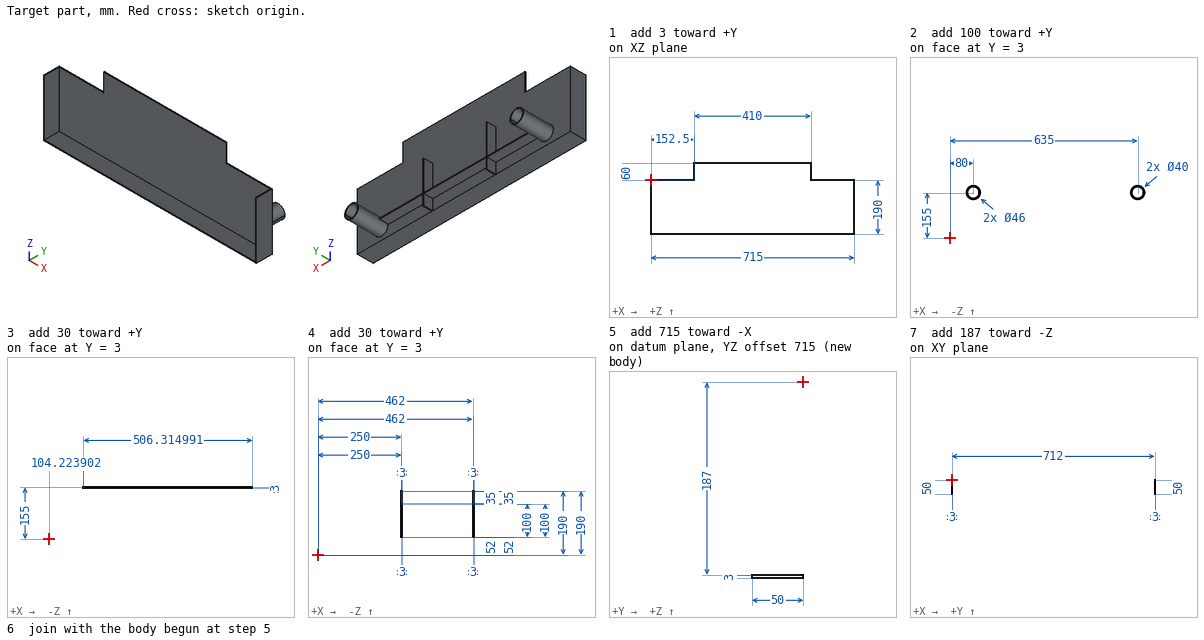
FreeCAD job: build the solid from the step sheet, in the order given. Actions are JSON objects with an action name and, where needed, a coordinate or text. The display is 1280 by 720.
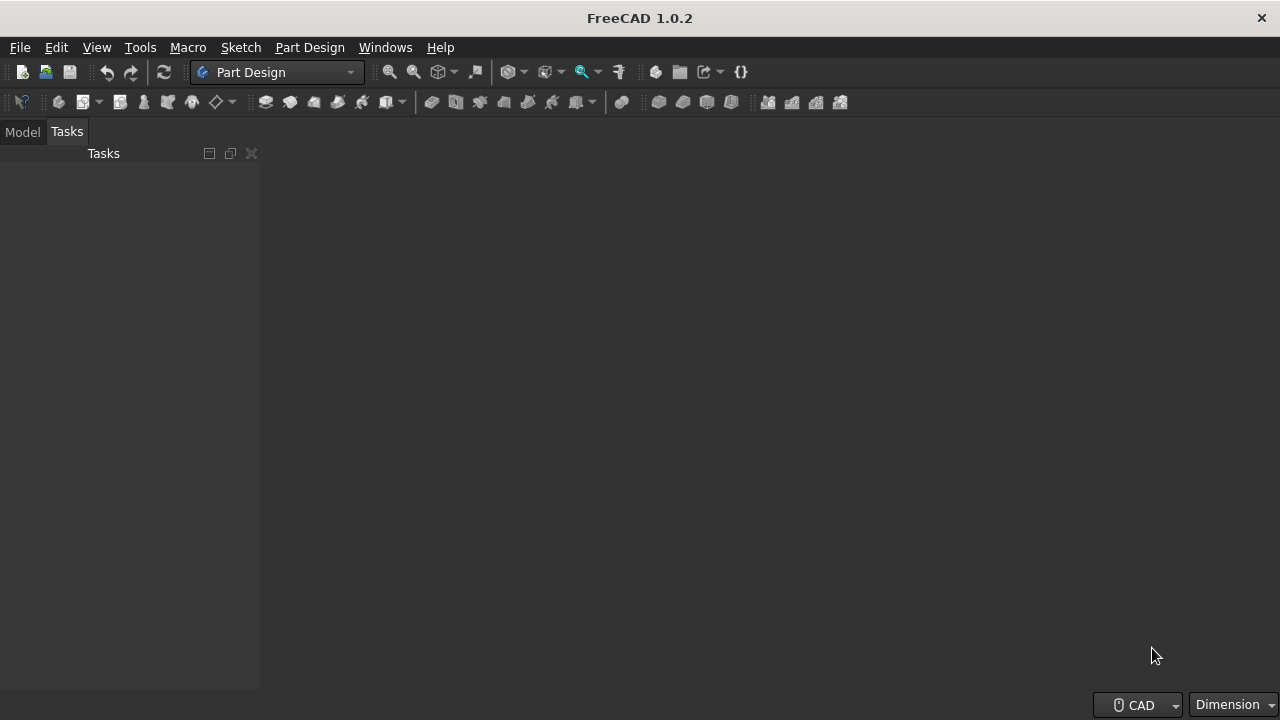
{"action": "left_click", "coordinate": [22, 72]}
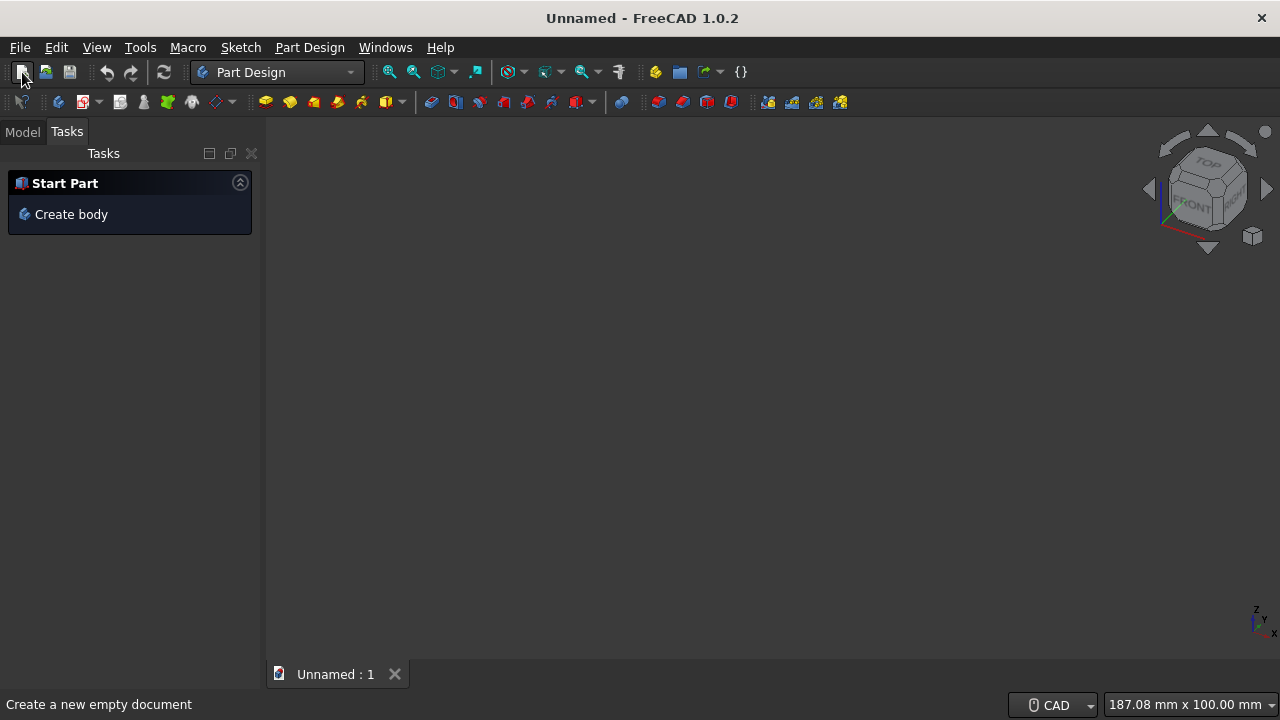
{"action": "left_click", "coordinate": [84, 102]}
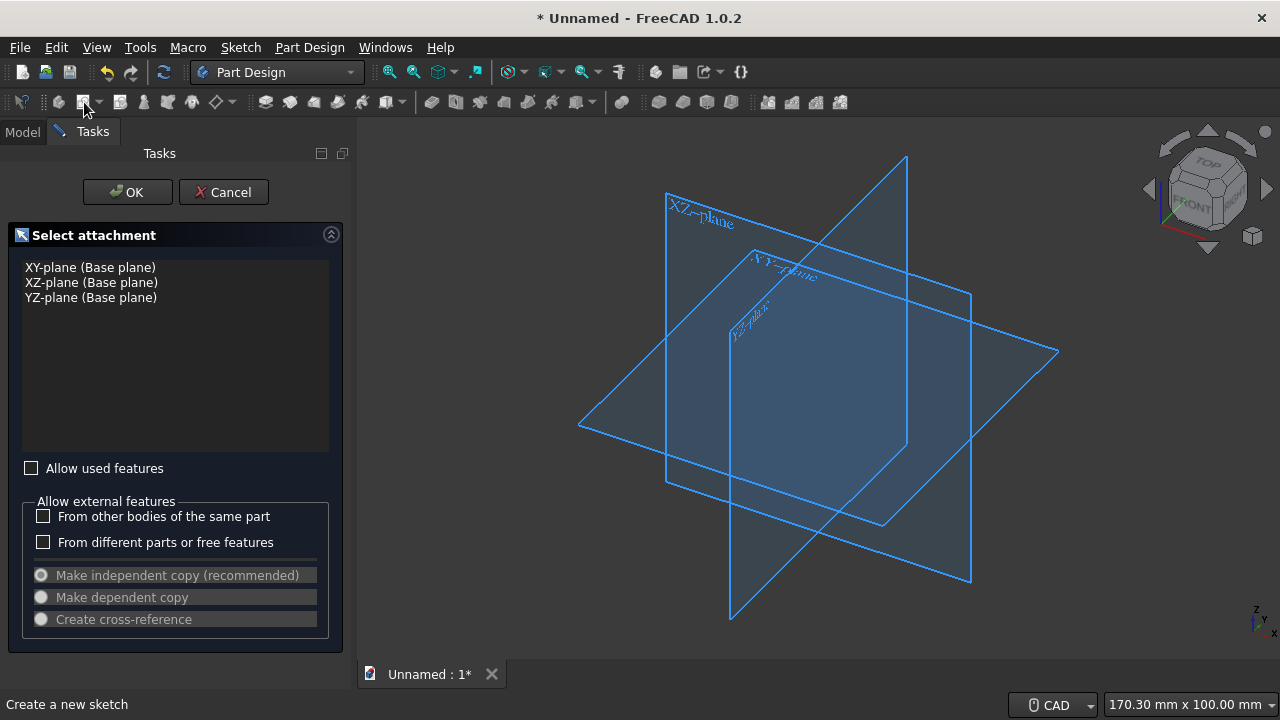
{"action": "left_click", "coordinate": [82, 282]}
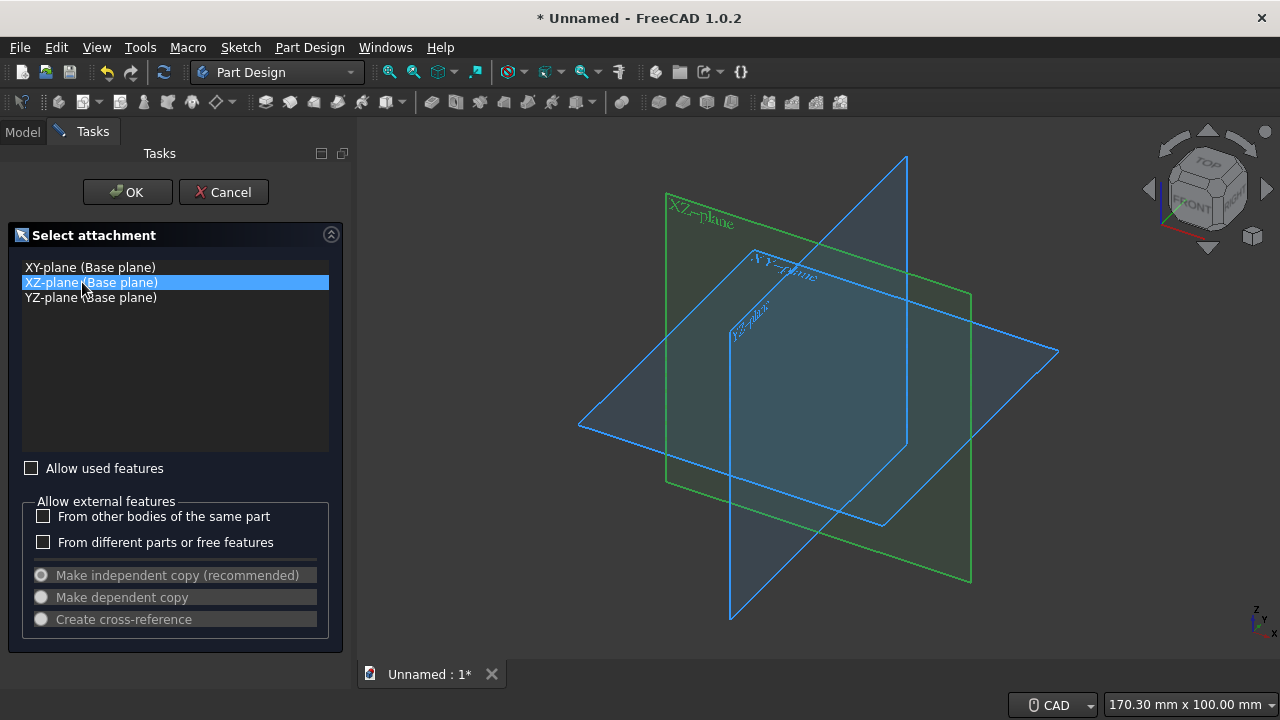
{"action": "left_click", "coordinate": [128, 192]}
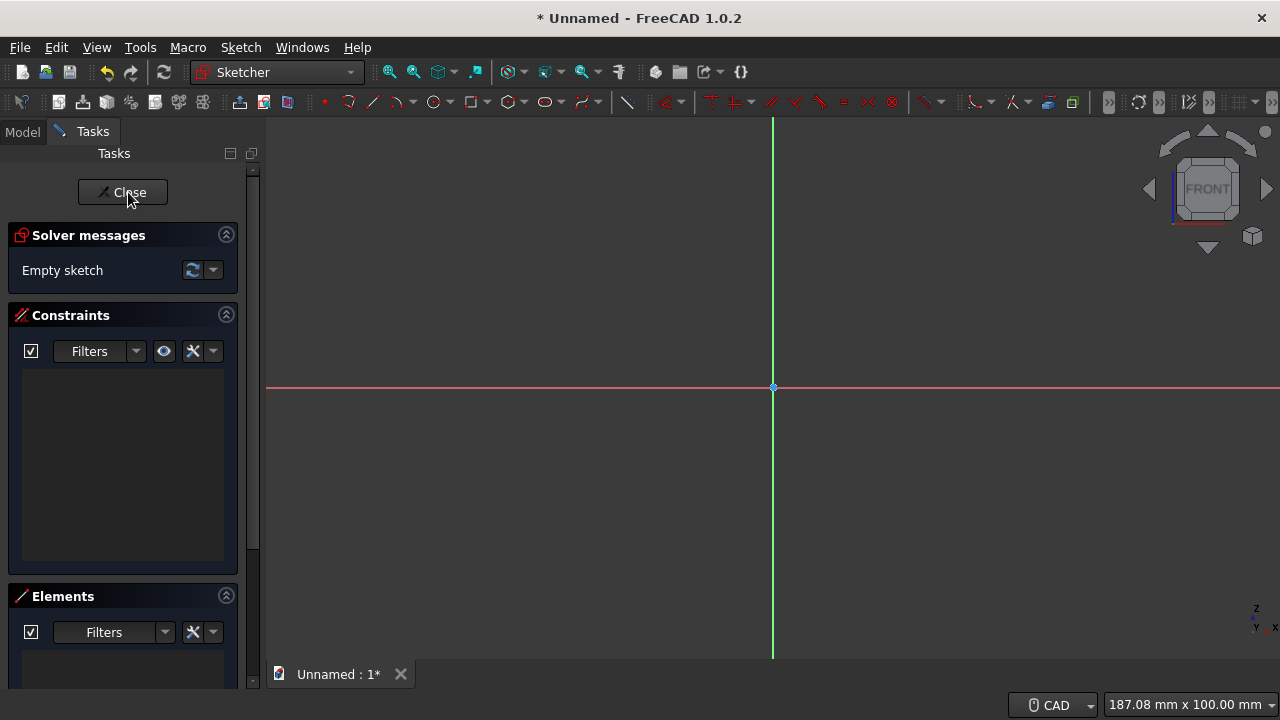
{"action": "scroll", "coordinate": [391, 333], "scroll_direction": "down", "scroll_amount": 10}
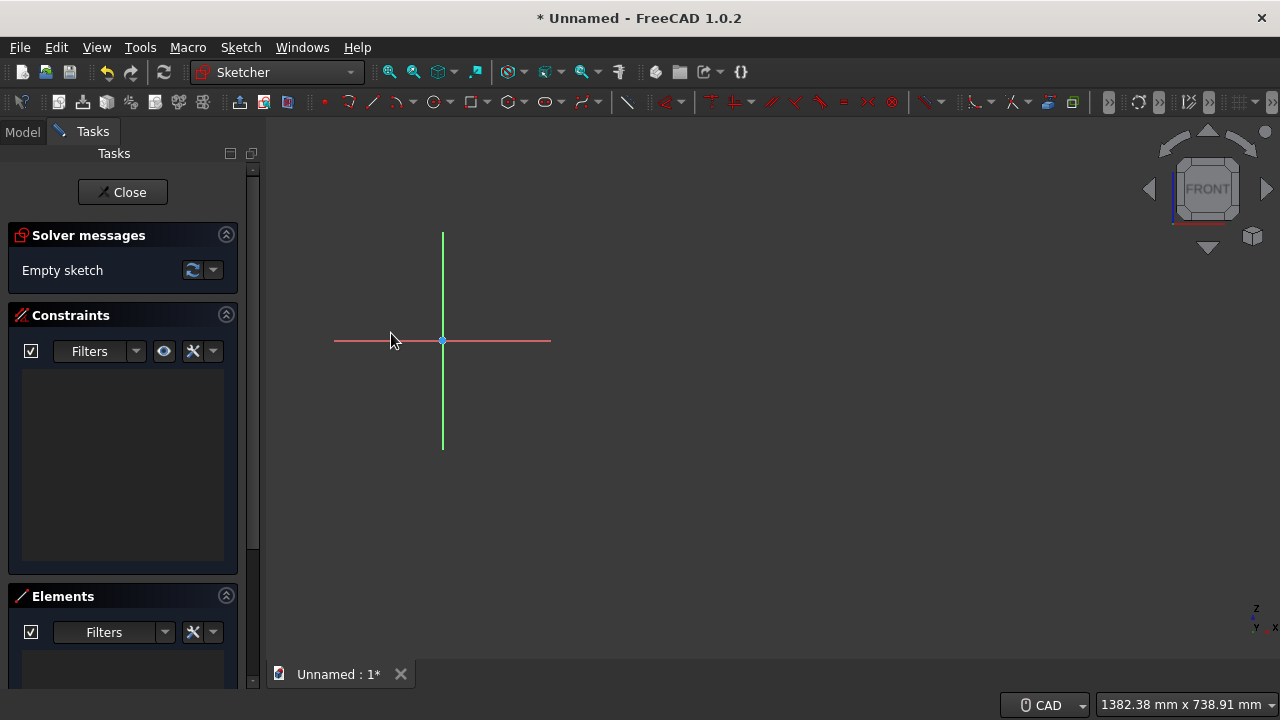
{"action": "key", "text": "g m"}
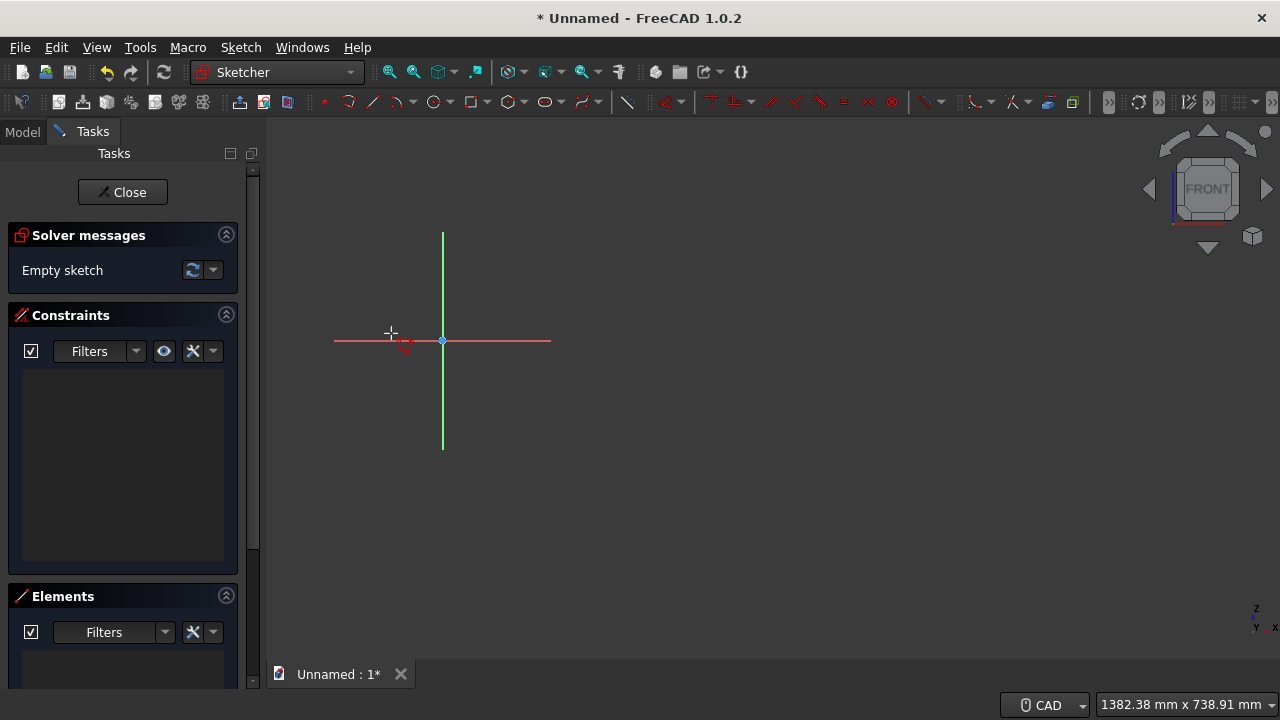
{"action": "left_click", "coordinate": [443, 341]}
{"action": "left_click", "coordinate": [555, 350]}
{"action": "left_click", "coordinate": [555, 297]}
{"action": "left_click", "coordinate": [855, 297]}
{"action": "left_click", "coordinate": [855, 341]}
{"action": "left_click", "coordinate": [967, 350]}
{"action": "left_click", "coordinate": [967, 480]}
{"action": "left_click", "coordinate": [452, 480]}
{"action": "left_click", "coordinate": [443, 341]}
{"action": "key", "text": "Escape"}
{"action": "key", "text": "Escape"}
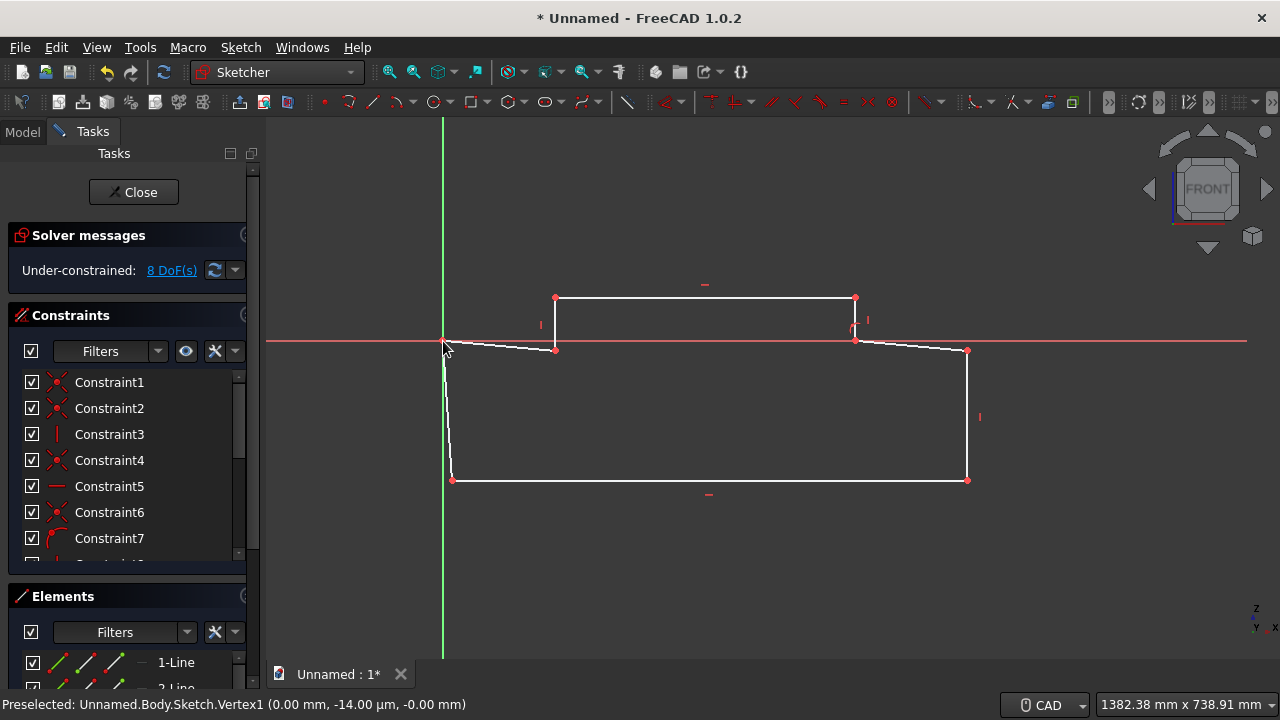
{"action": "left_click", "coordinate": [476, 344]}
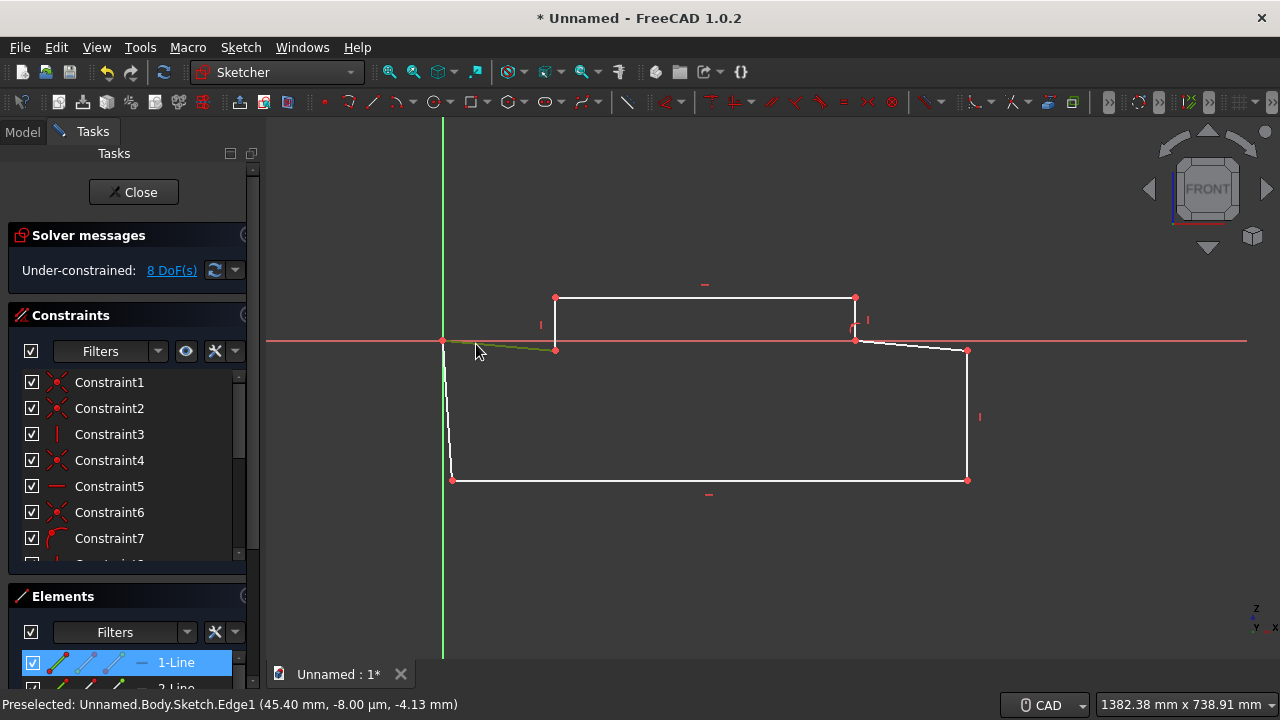
{"action": "left_click", "coordinate": [754, 102]}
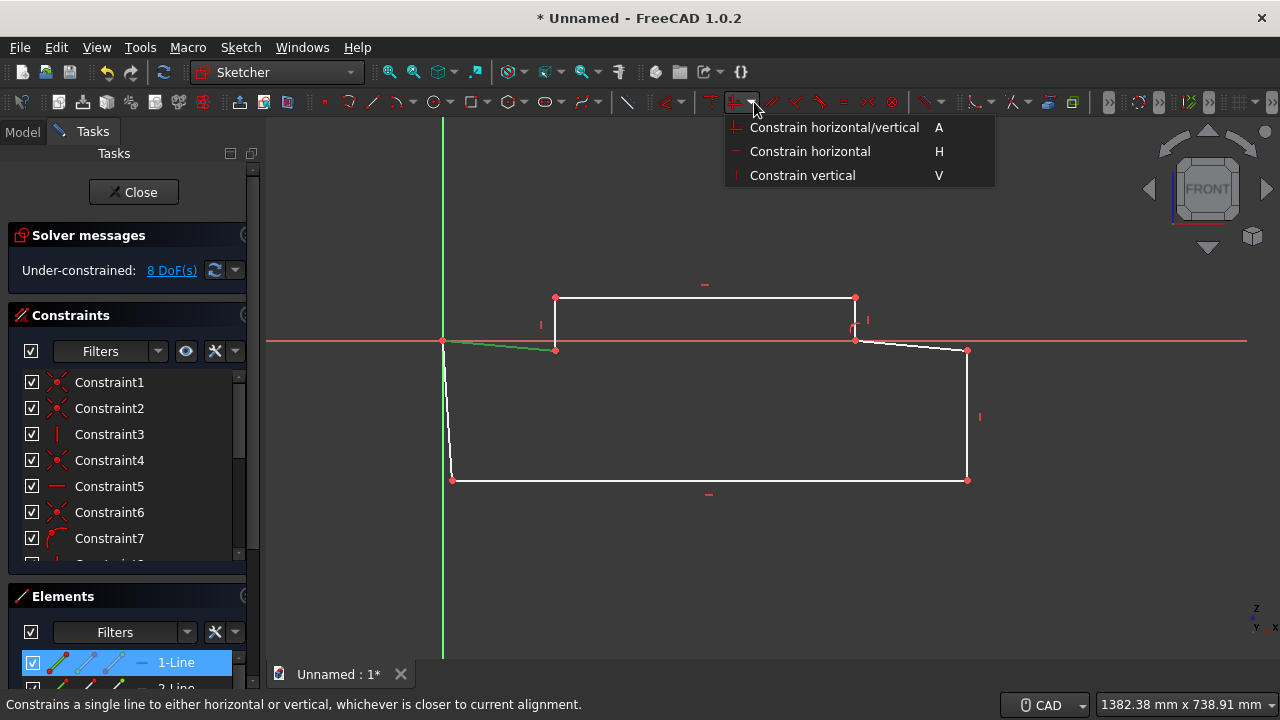
{"action": "left_click", "coordinate": [860, 151]}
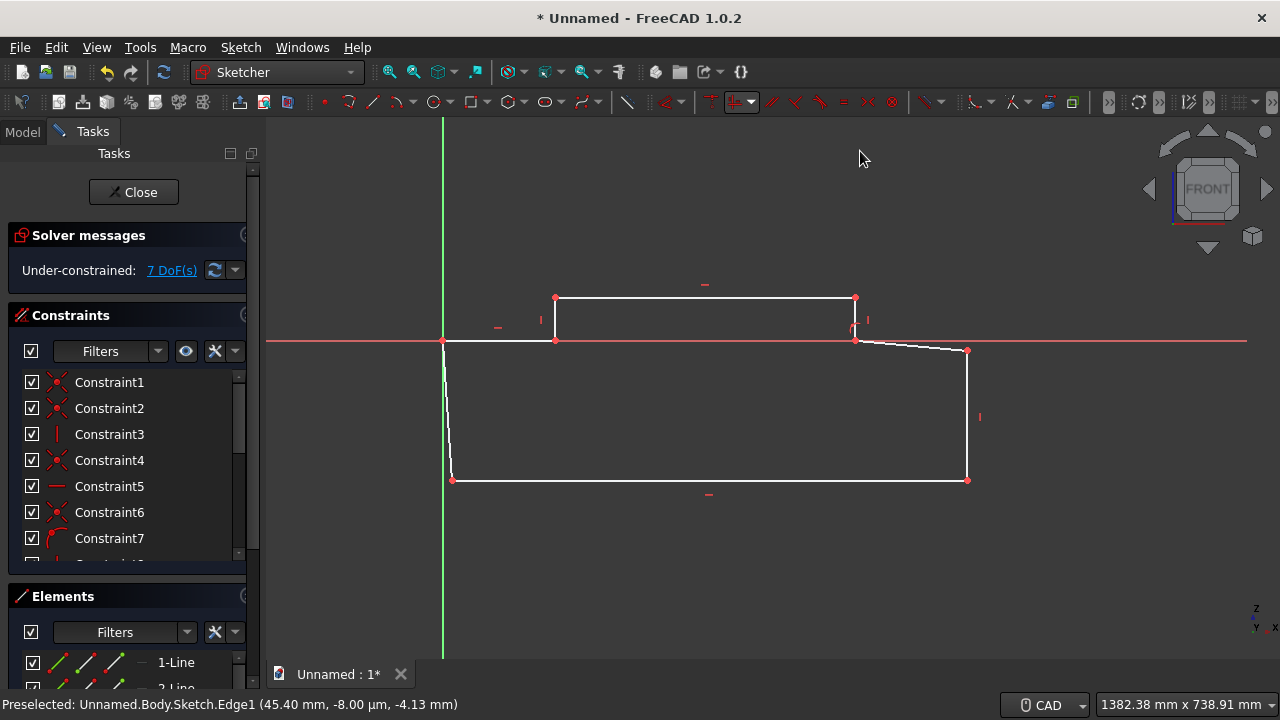
{"action": "left_click", "coordinate": [889, 344]}